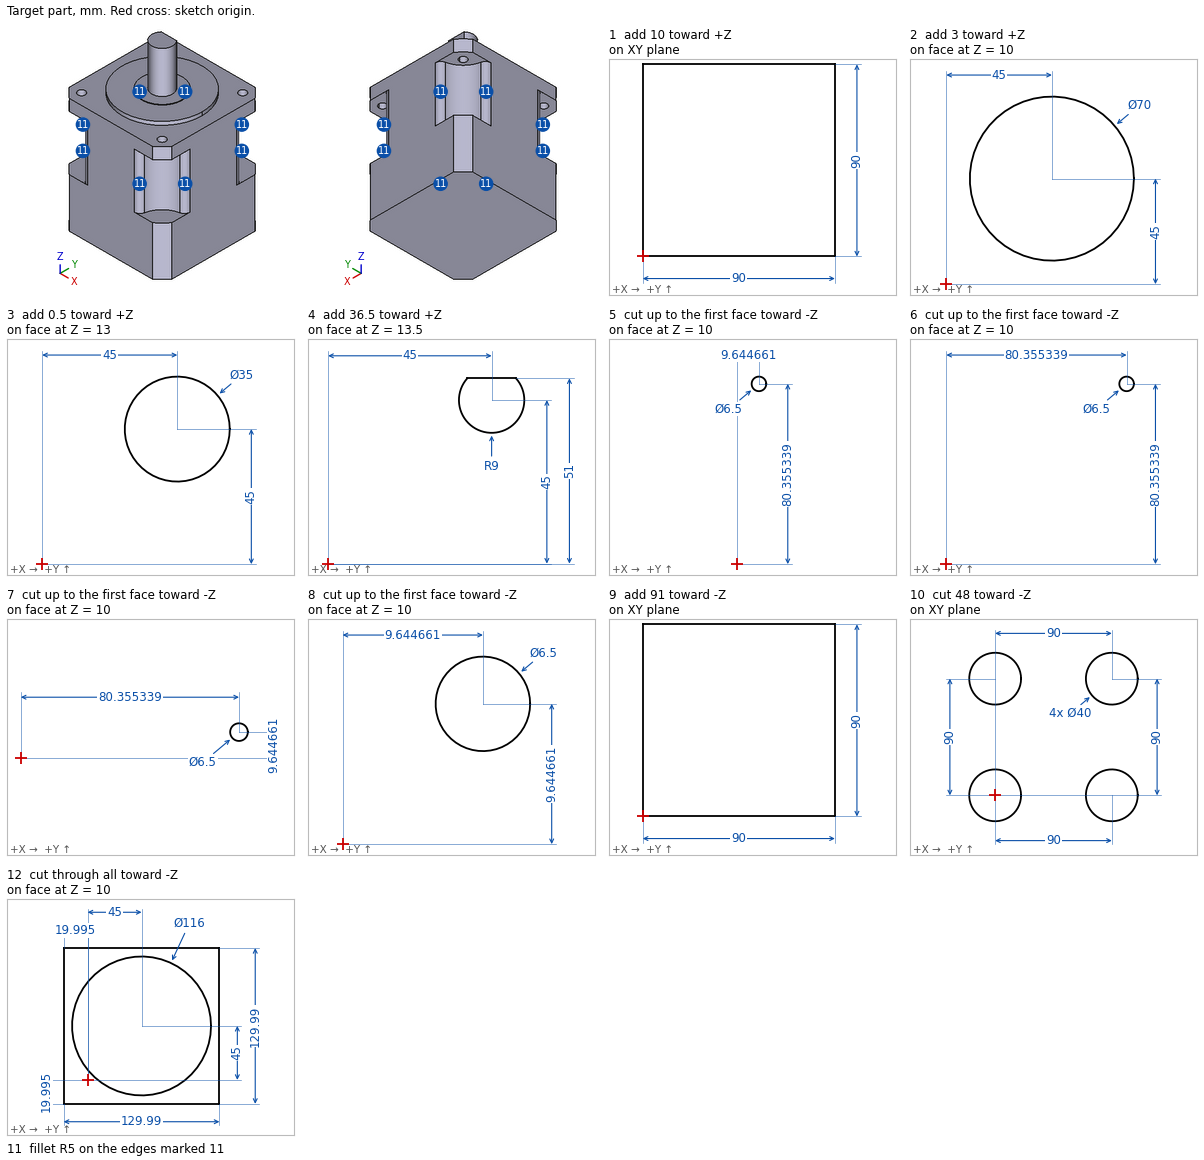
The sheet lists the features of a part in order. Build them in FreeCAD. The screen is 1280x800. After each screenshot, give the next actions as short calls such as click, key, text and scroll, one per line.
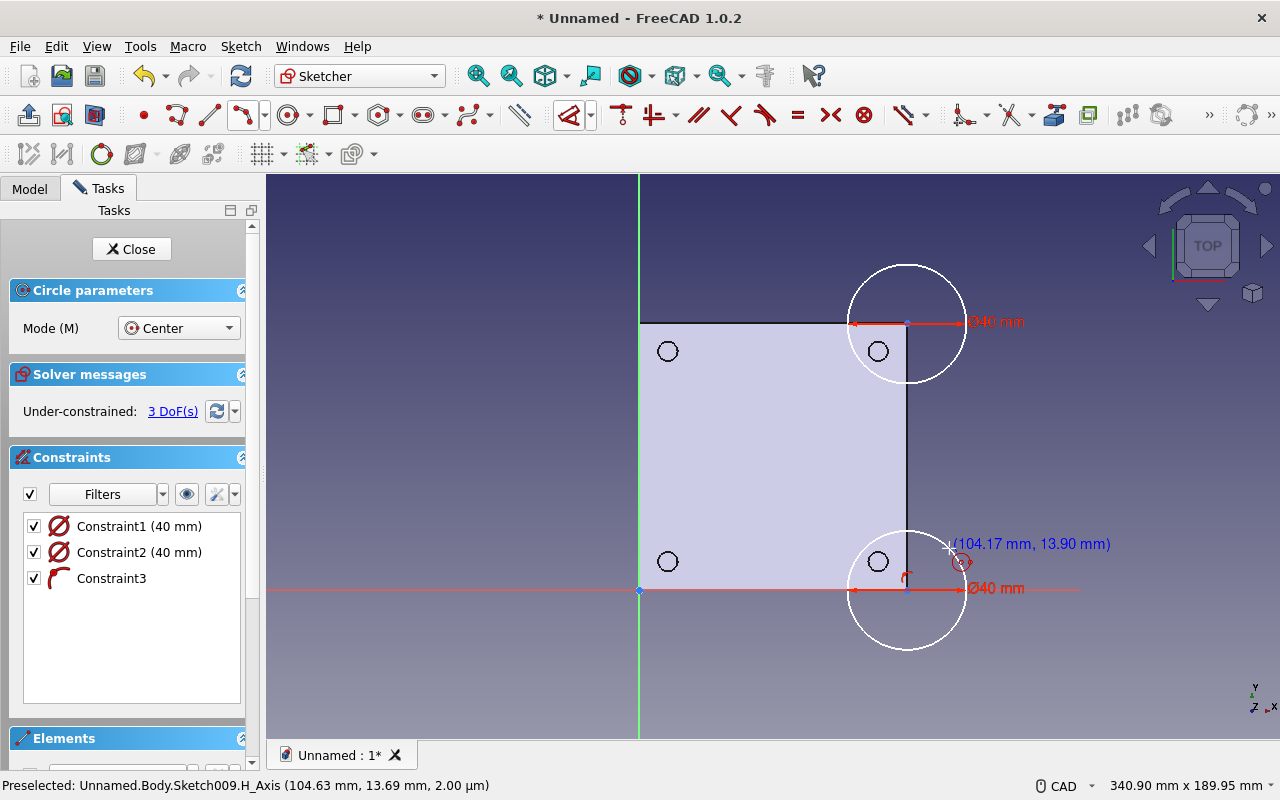
click(639, 590)
move(681, 548)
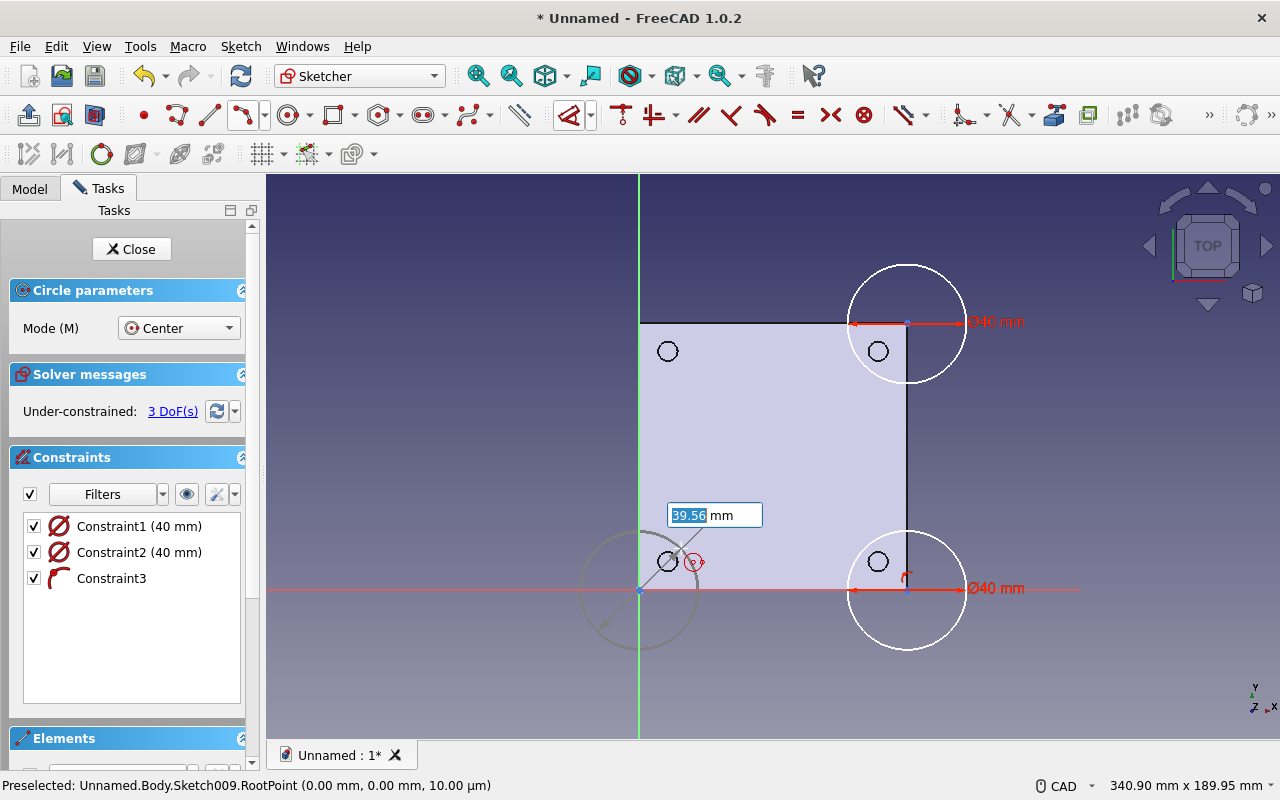
text(40)
key(Return)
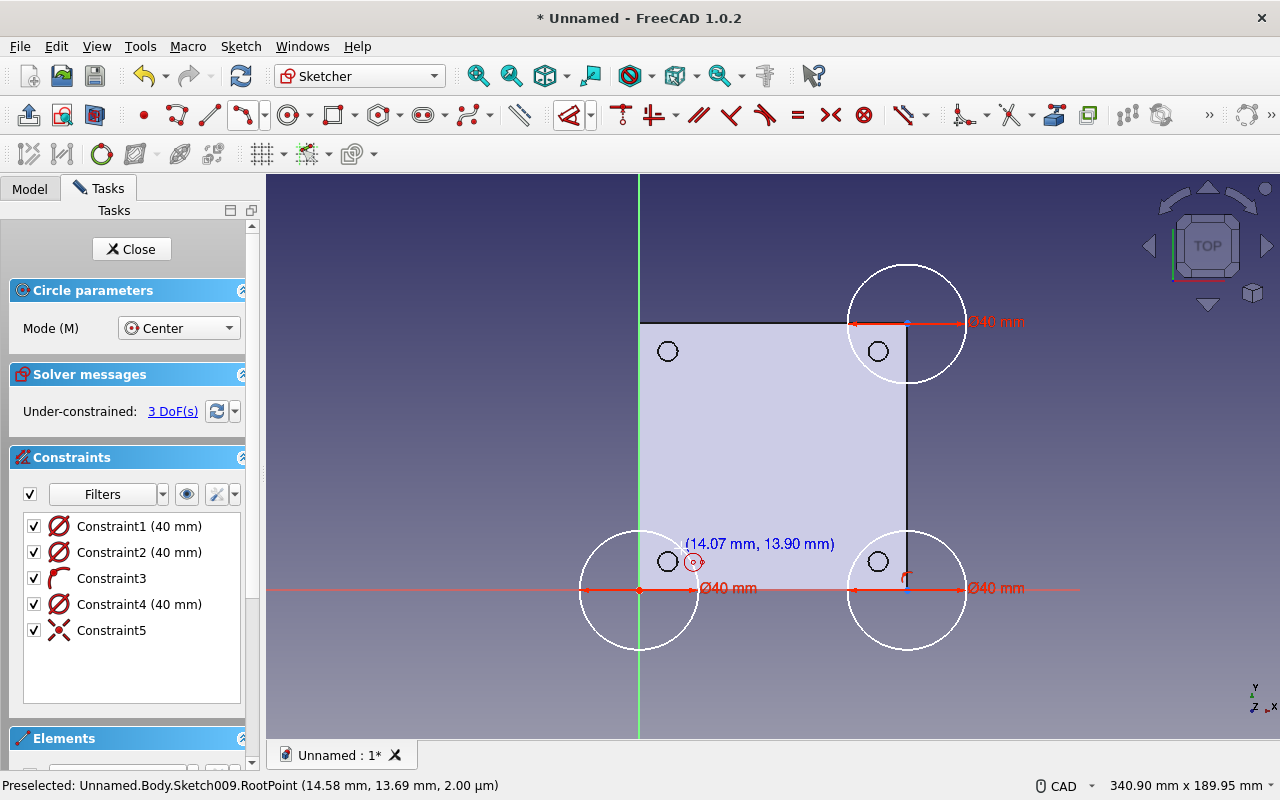
click(639, 323)
move(681, 281)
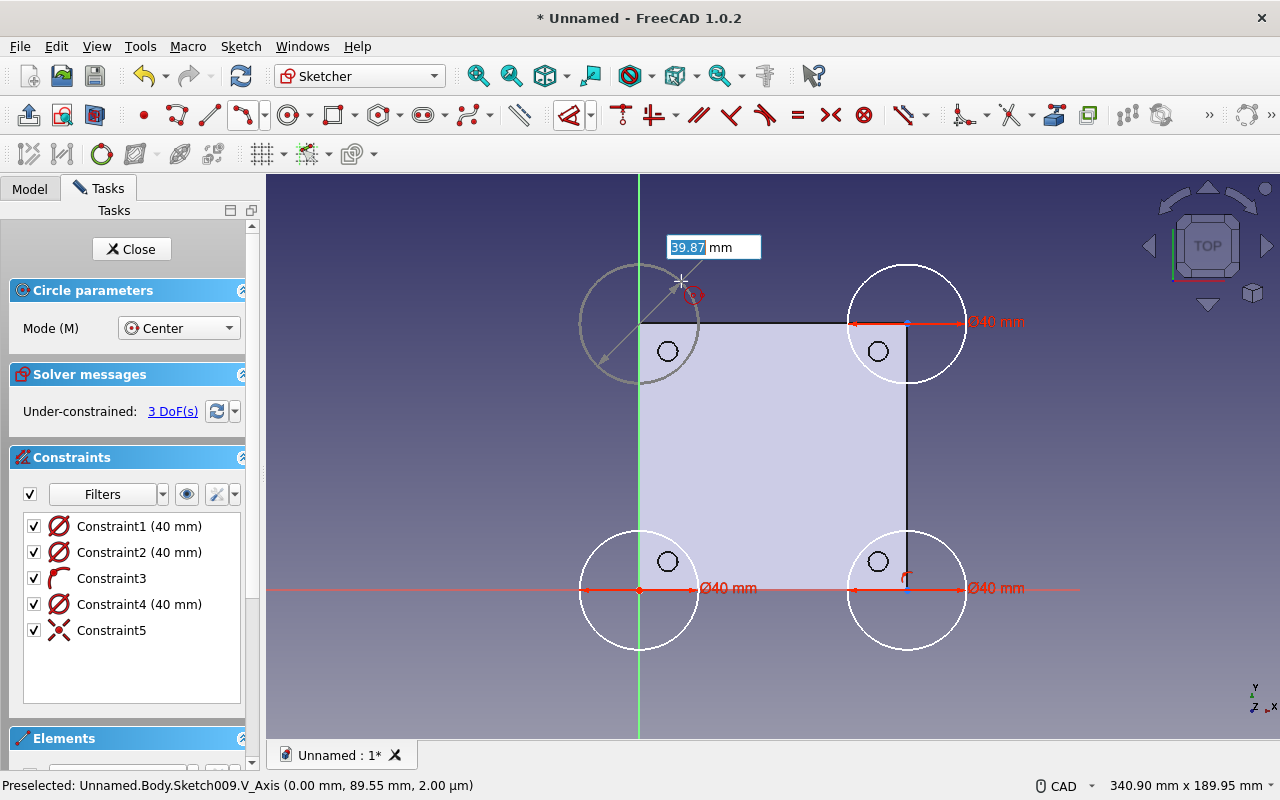
text(40)
key(Return)
key(Escape)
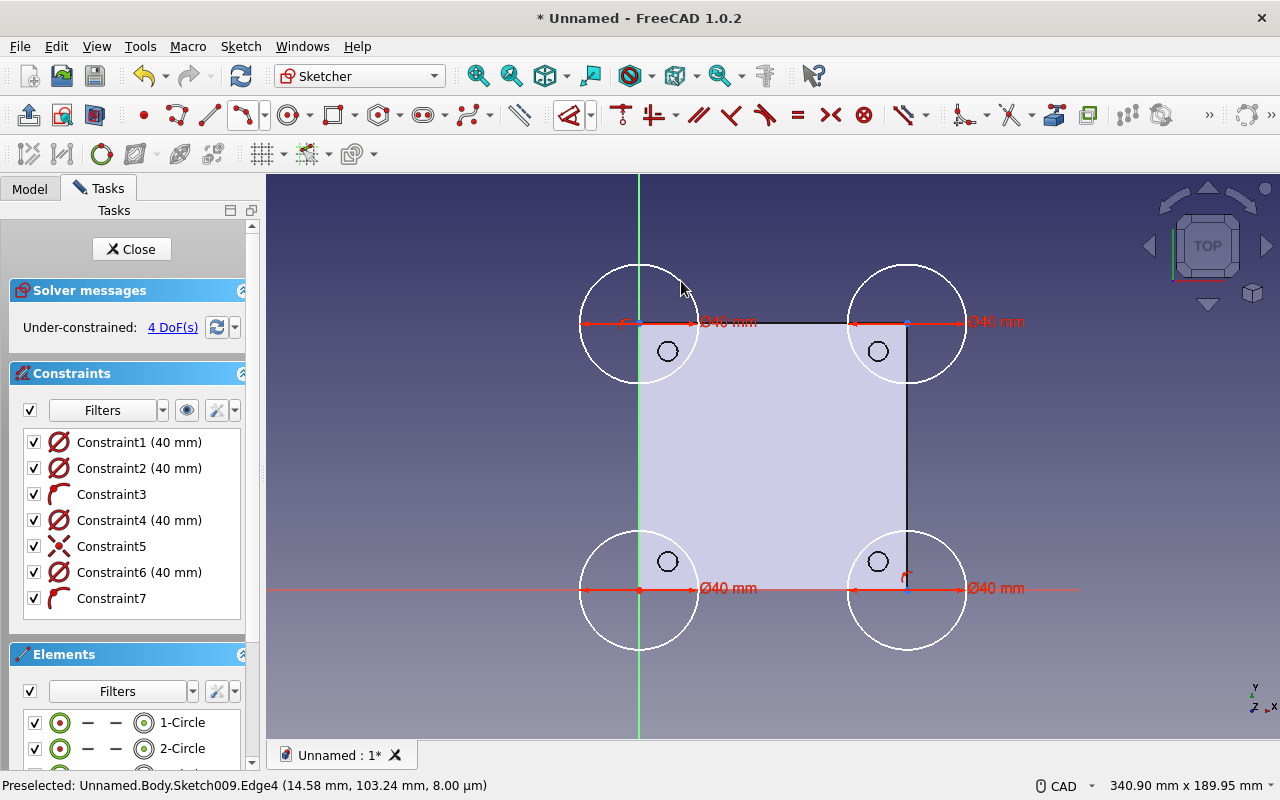
click(907, 324)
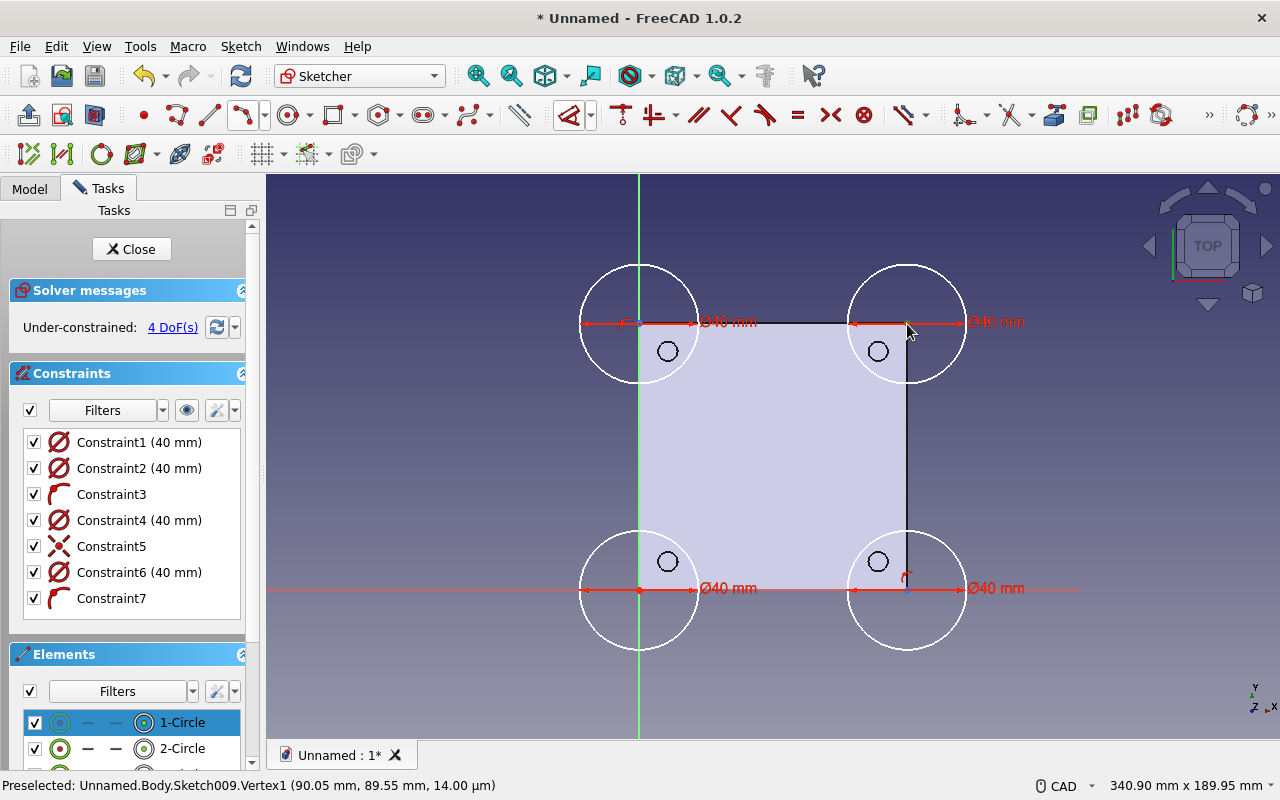
key(l)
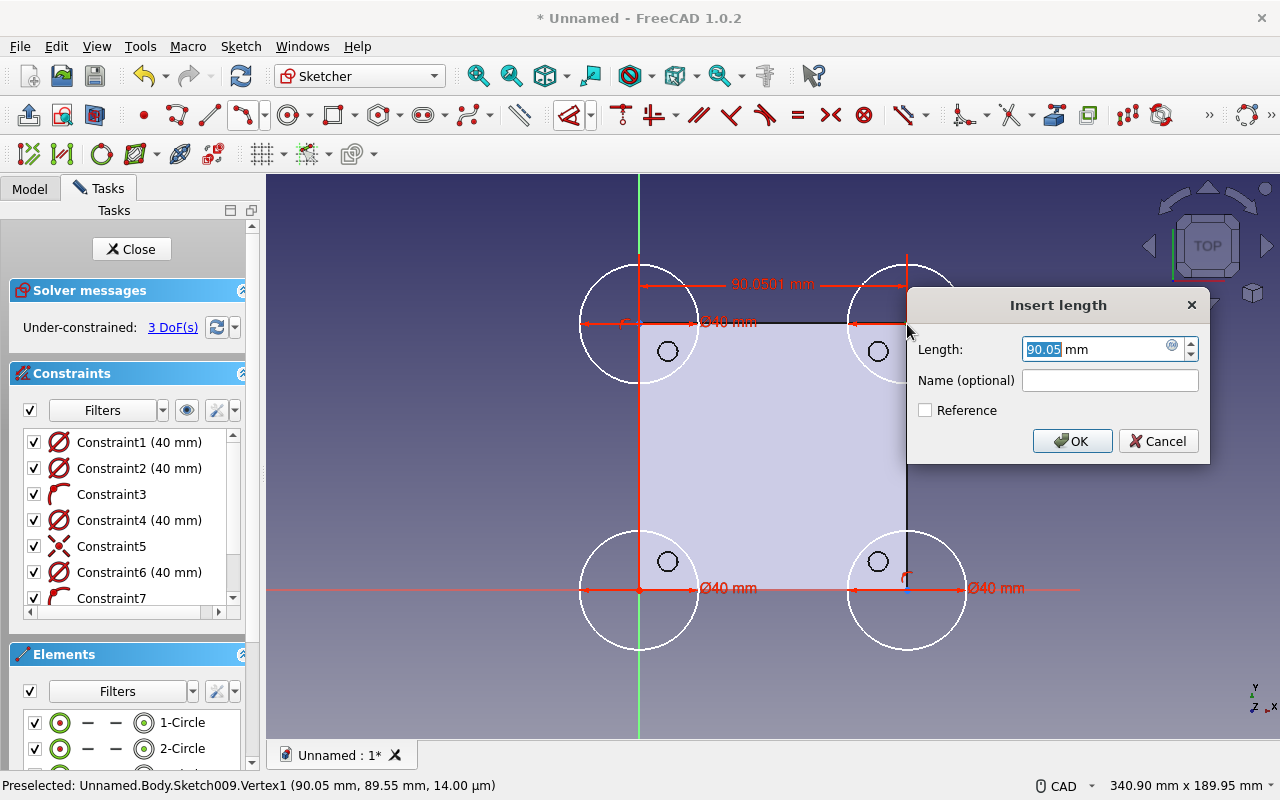
text(90)
key(Return)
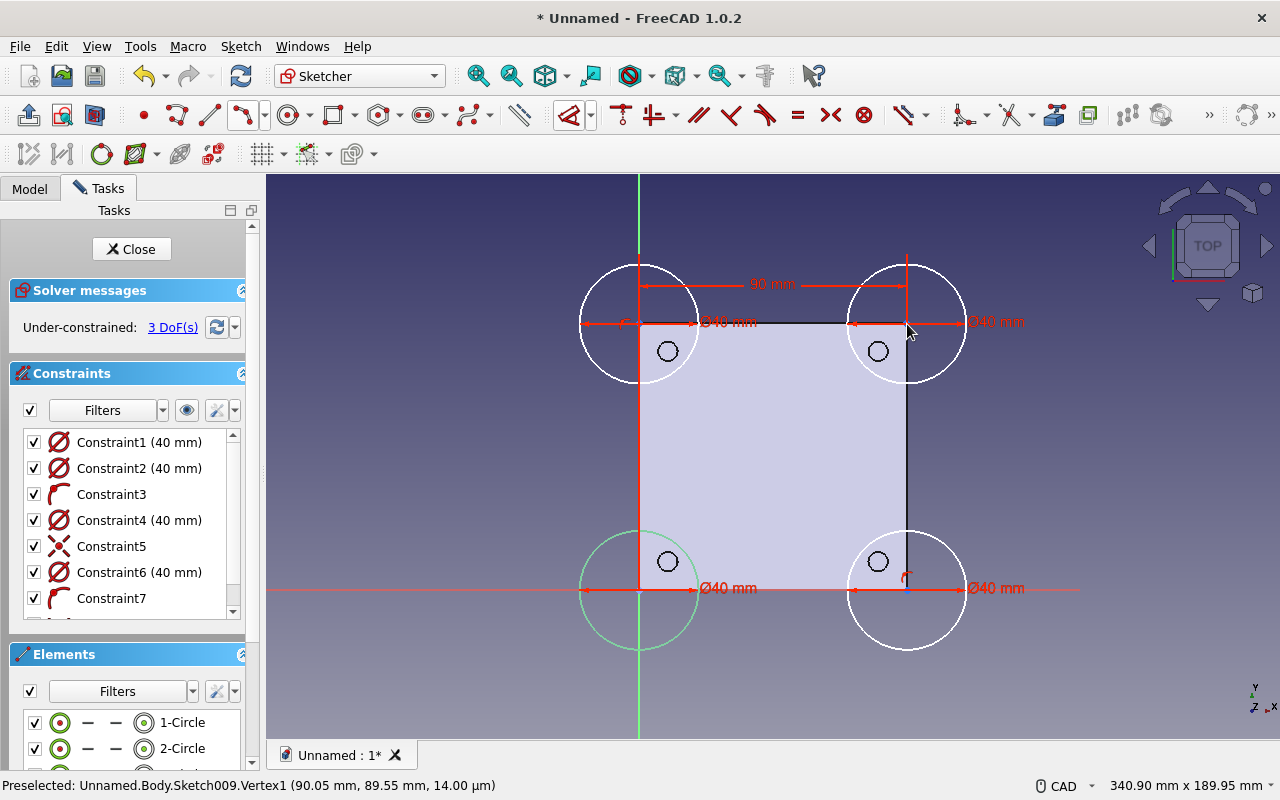
click(907, 324)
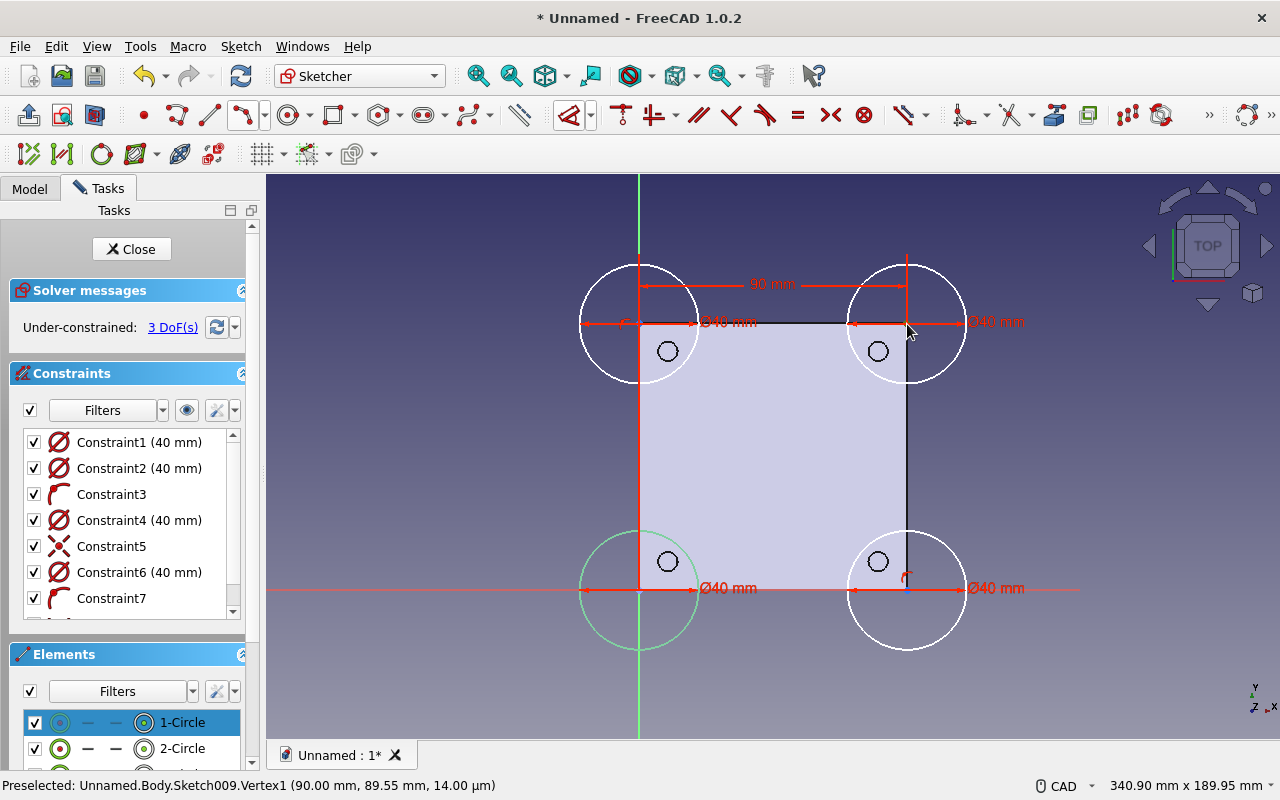
click(590, 116)